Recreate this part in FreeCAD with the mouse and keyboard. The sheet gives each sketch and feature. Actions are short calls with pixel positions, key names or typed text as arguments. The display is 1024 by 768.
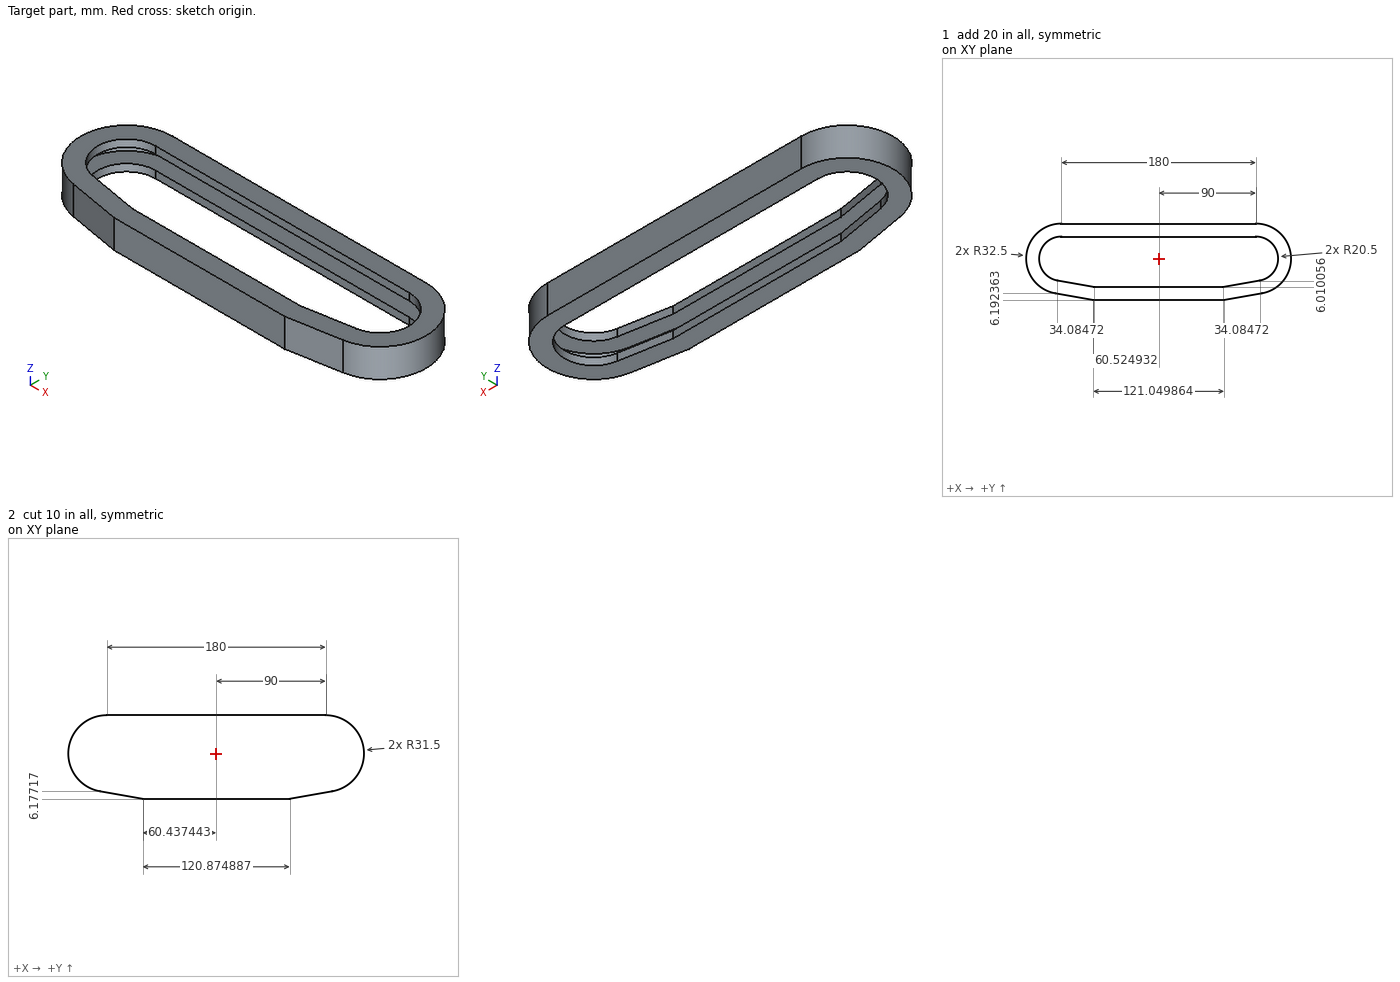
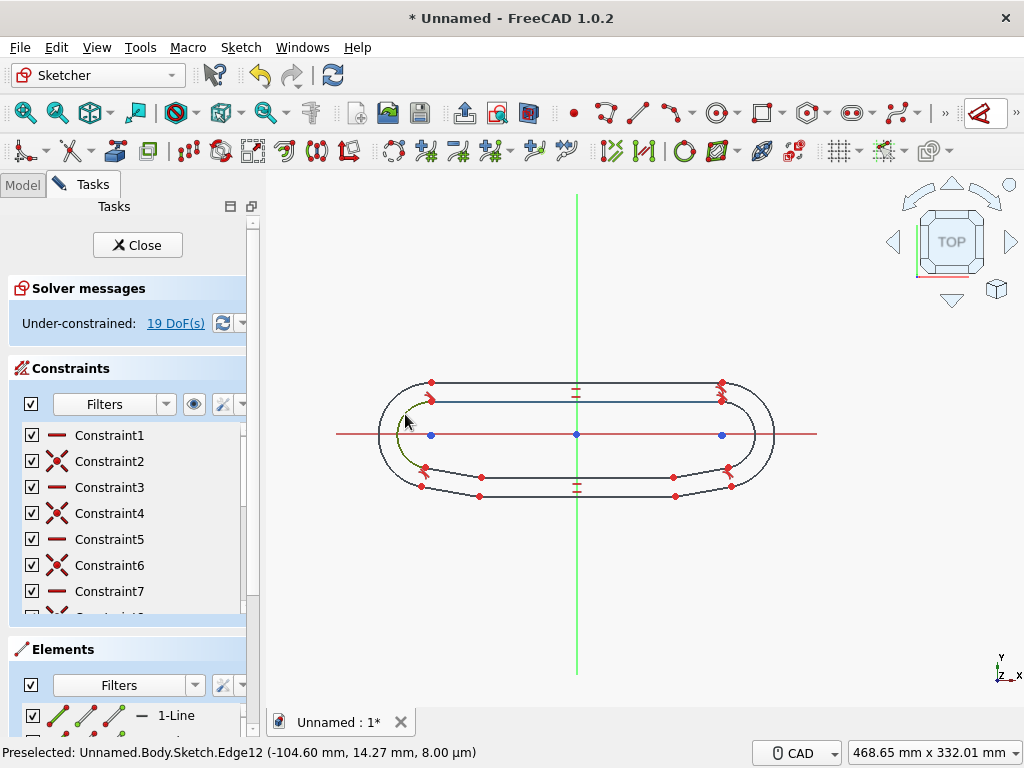
key(t)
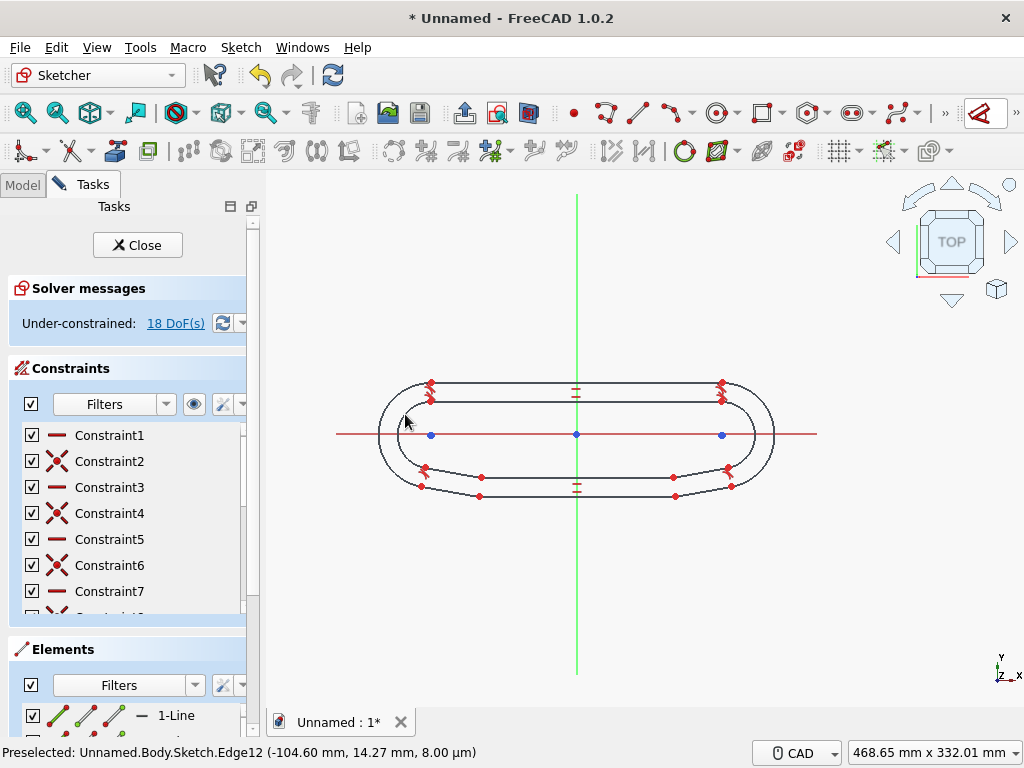
click(711, 471)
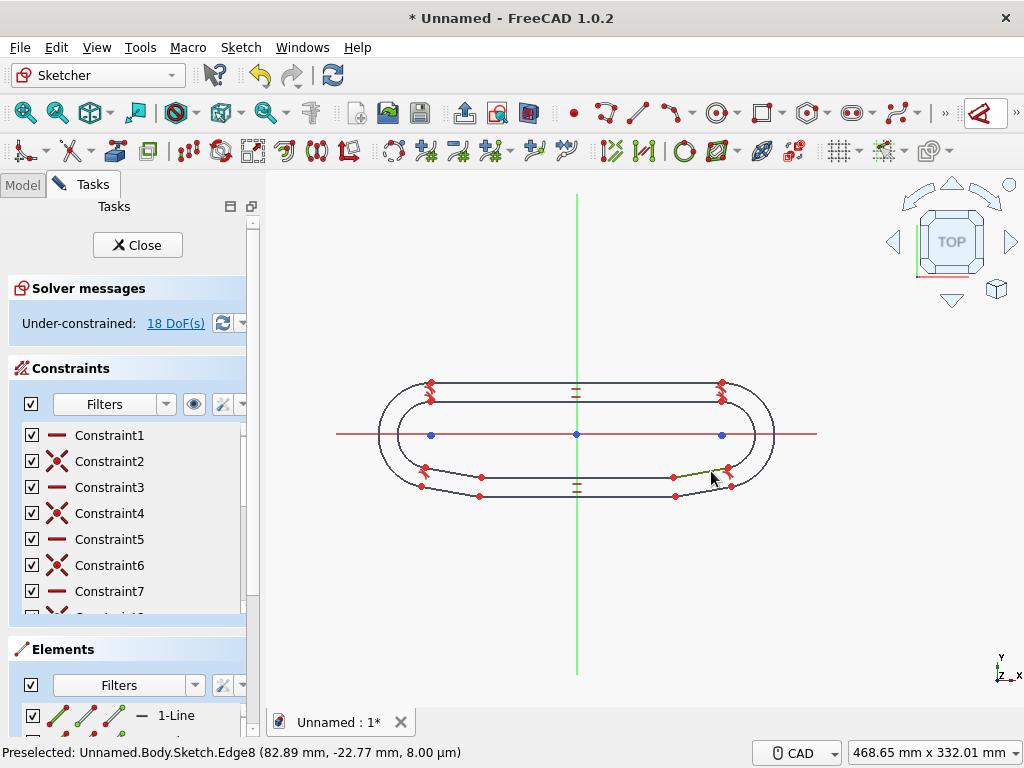
click(751, 451)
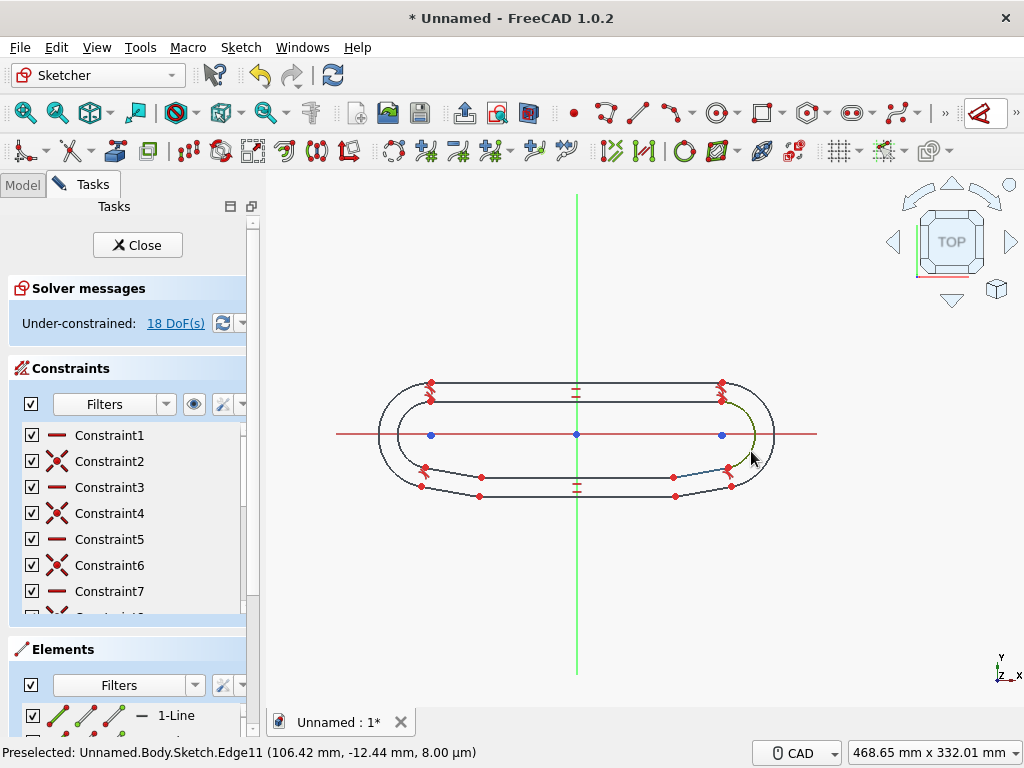
key(t)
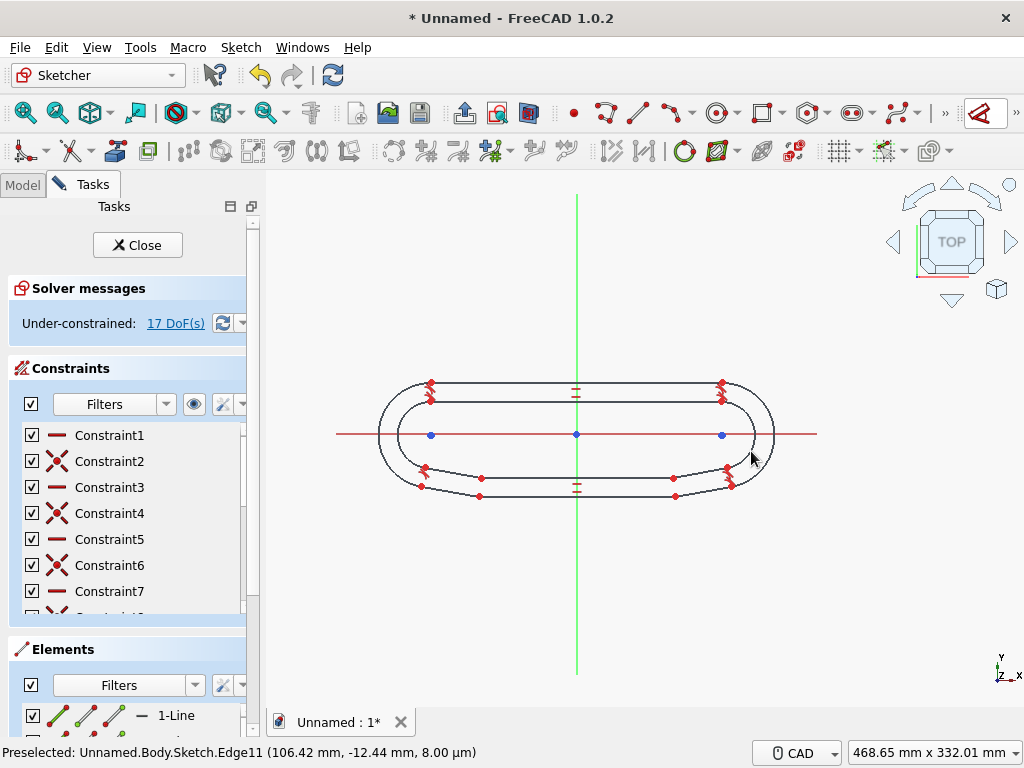
click(464, 475)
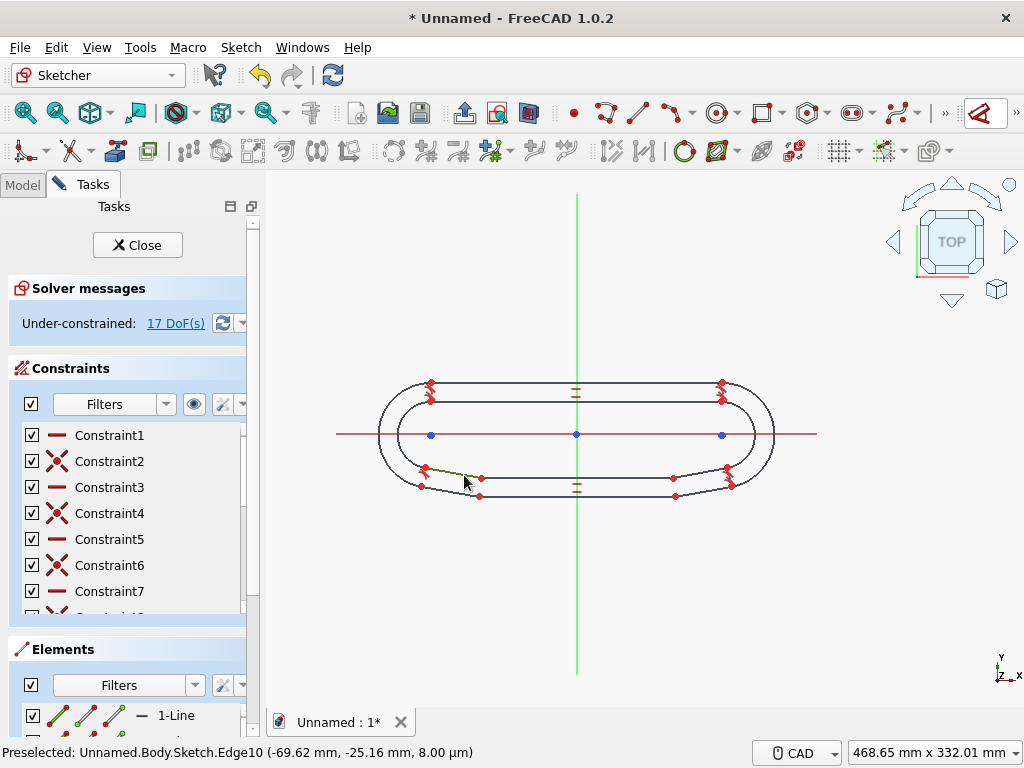
click(405, 414)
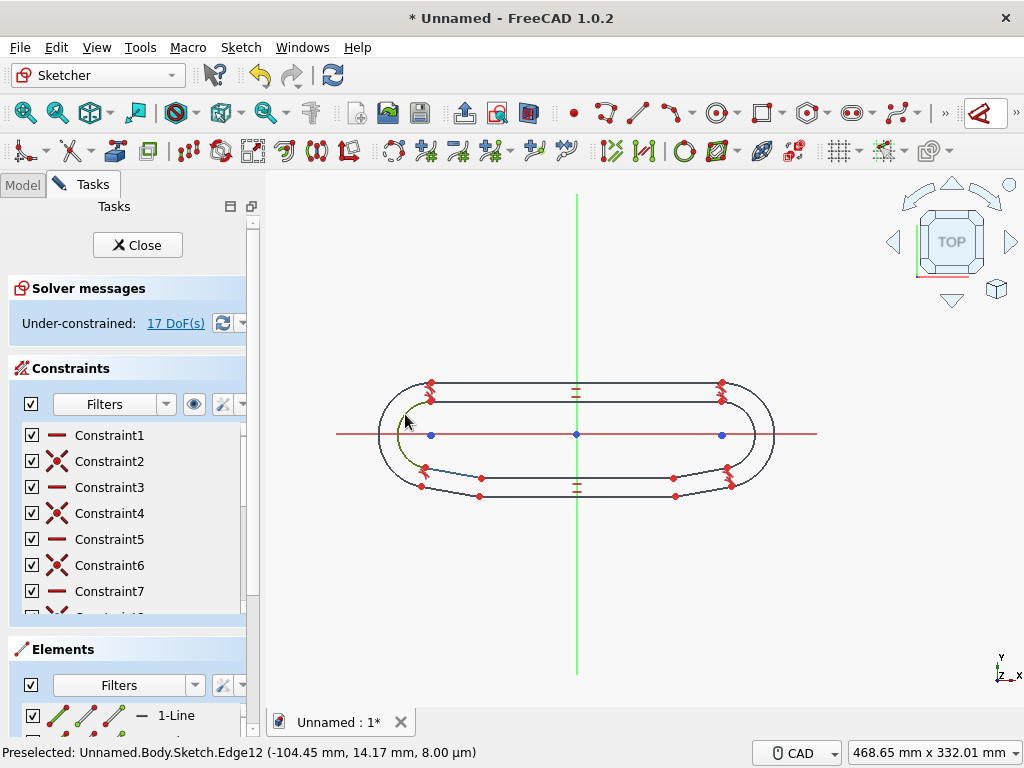
key(t)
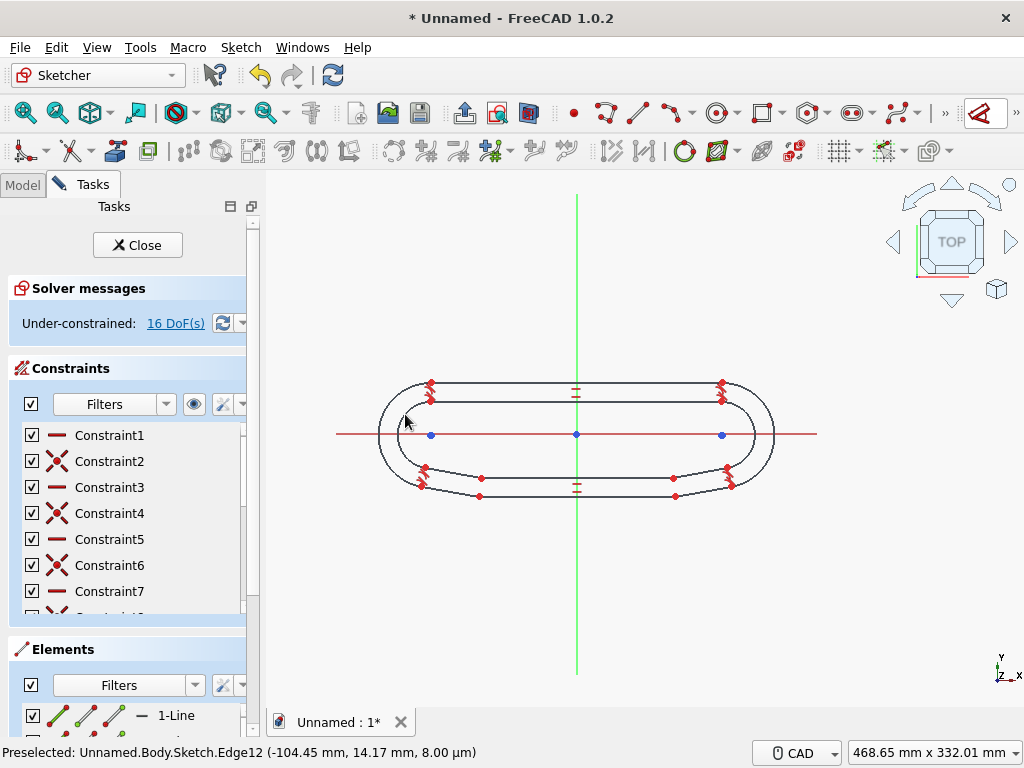
click(768, 461)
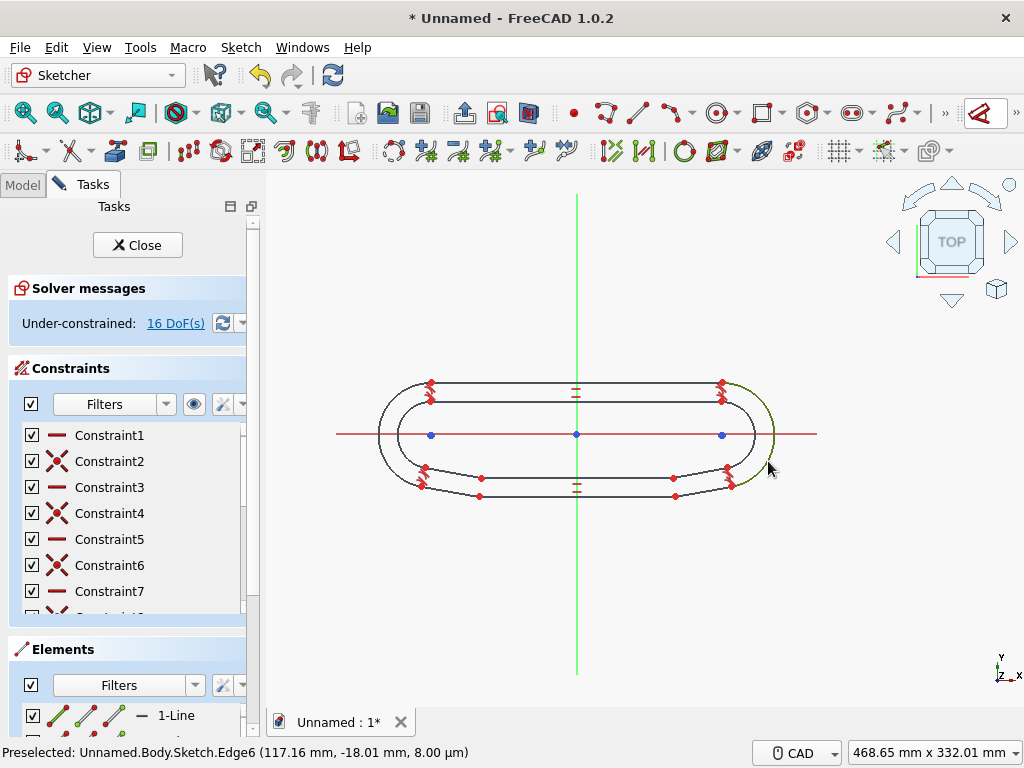
click(751, 451)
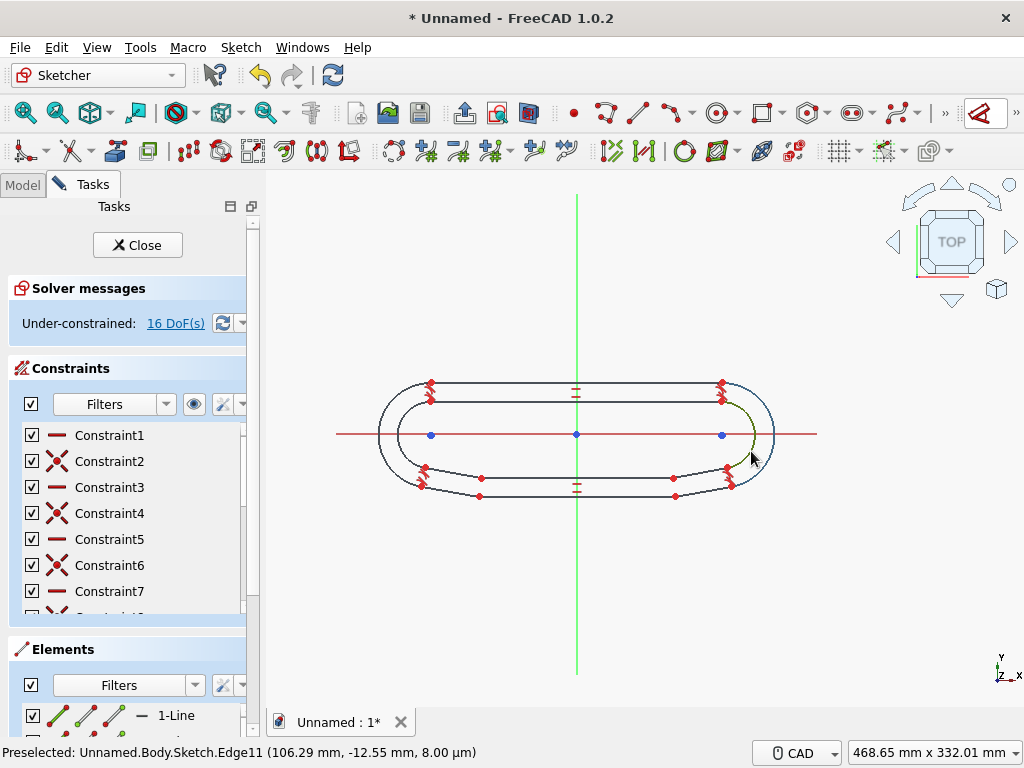
key(c)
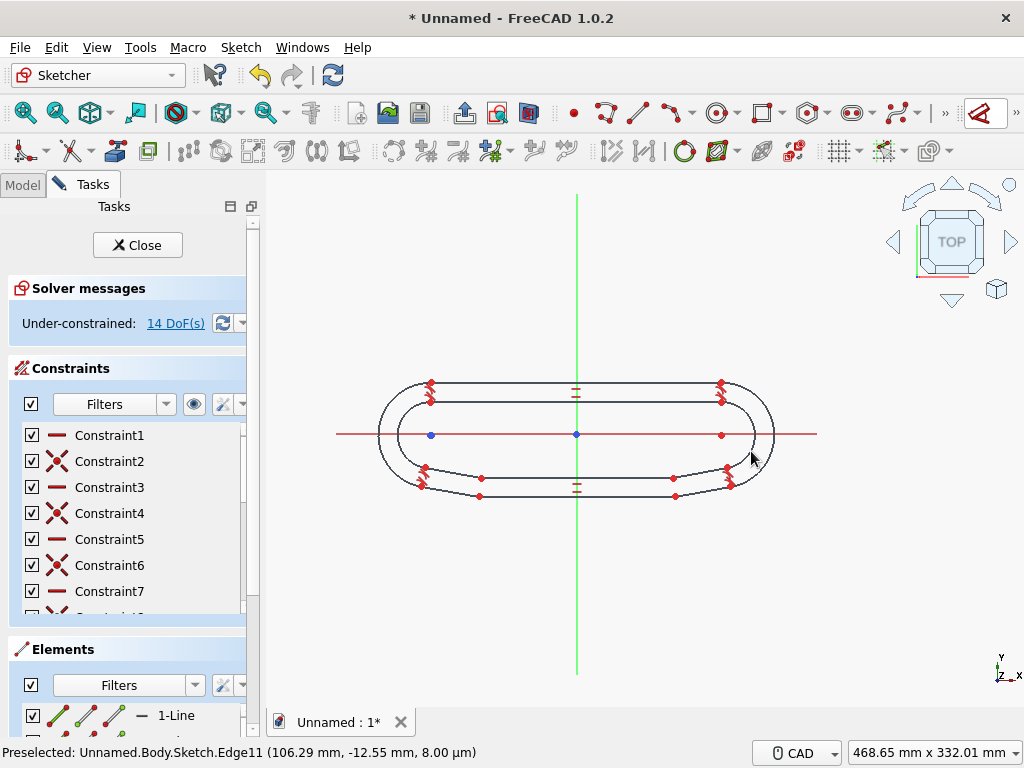
click(390, 402)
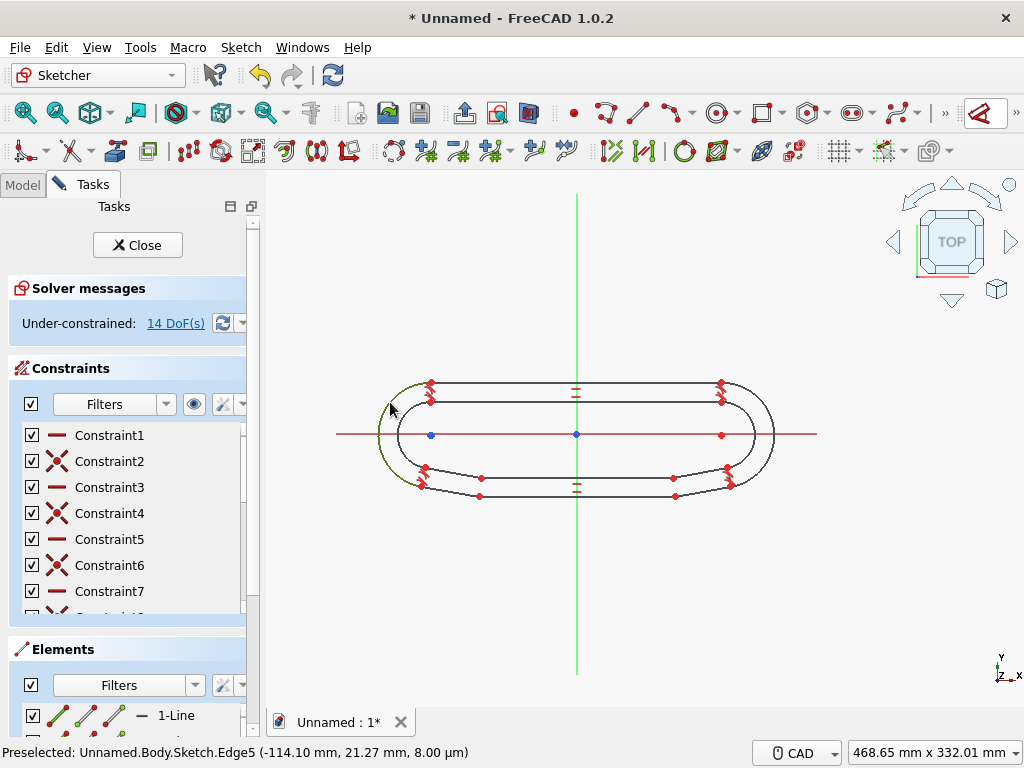
click(405, 414)